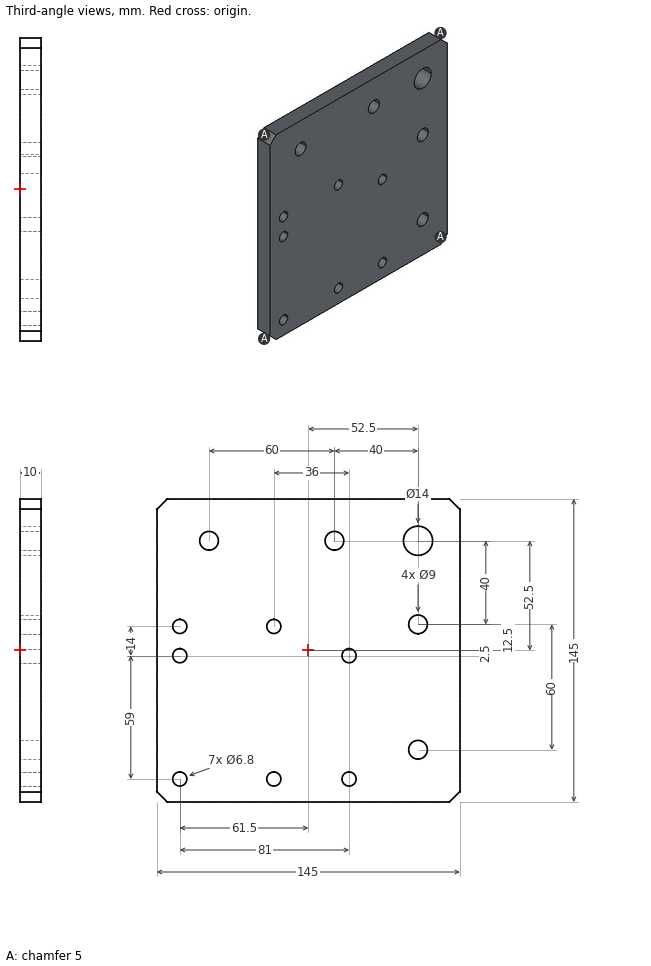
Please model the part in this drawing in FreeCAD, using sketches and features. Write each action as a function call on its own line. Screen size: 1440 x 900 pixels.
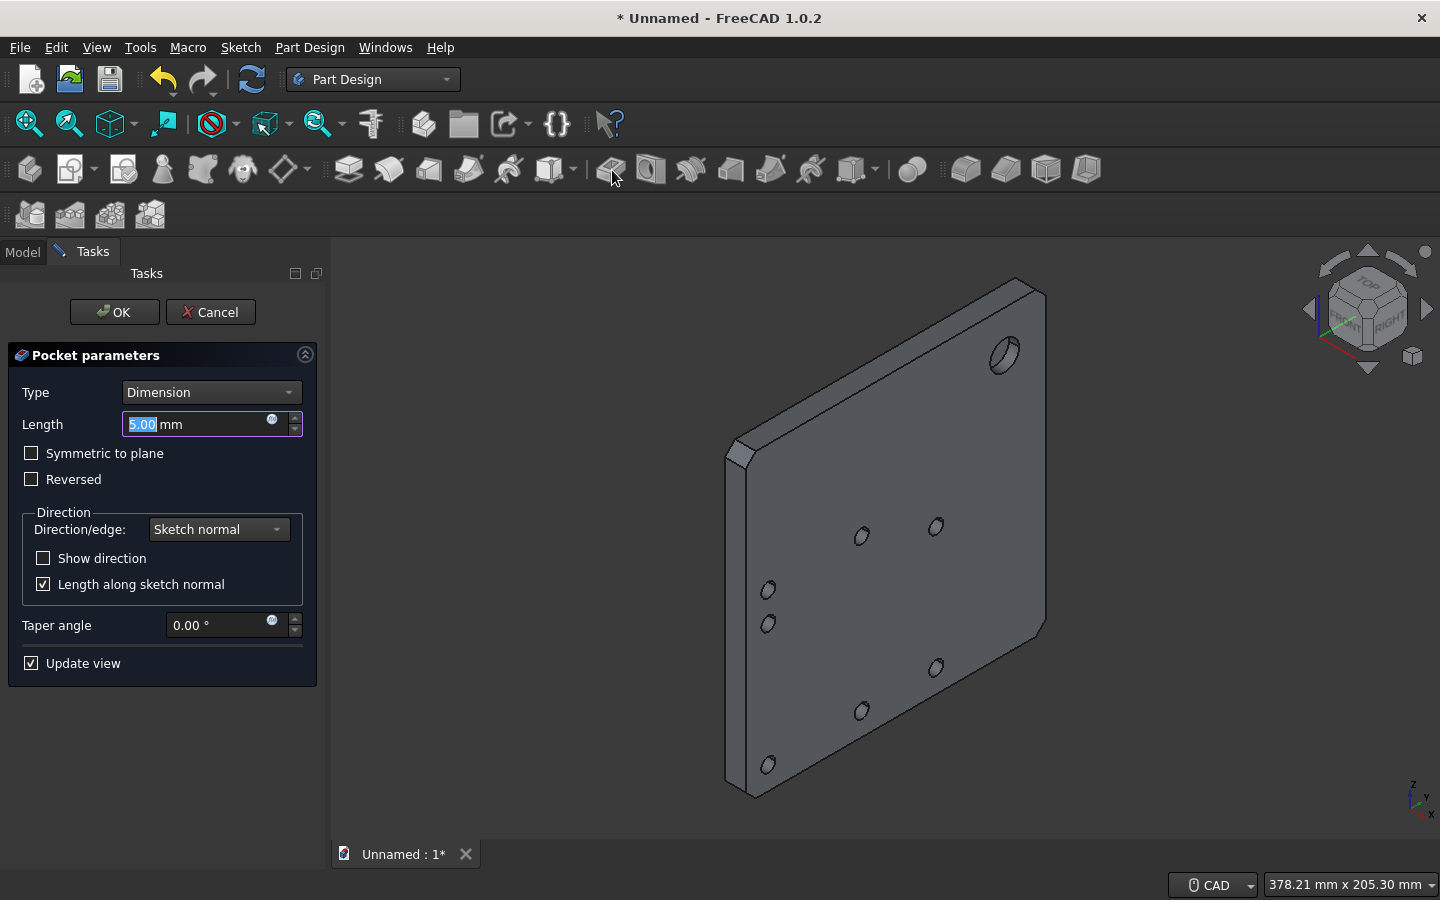
click(212, 392)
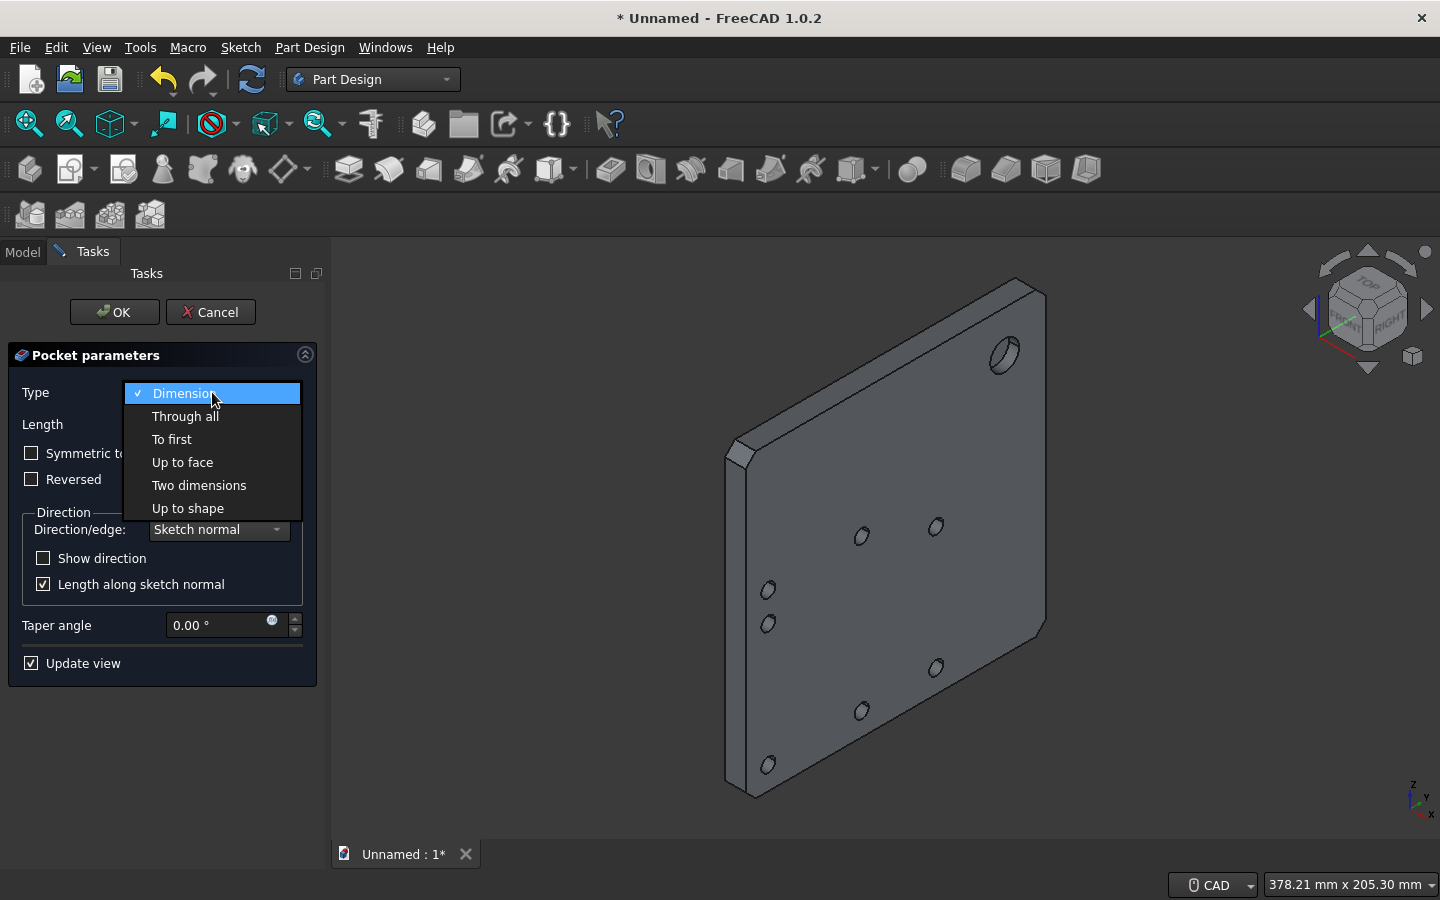
click(212, 416)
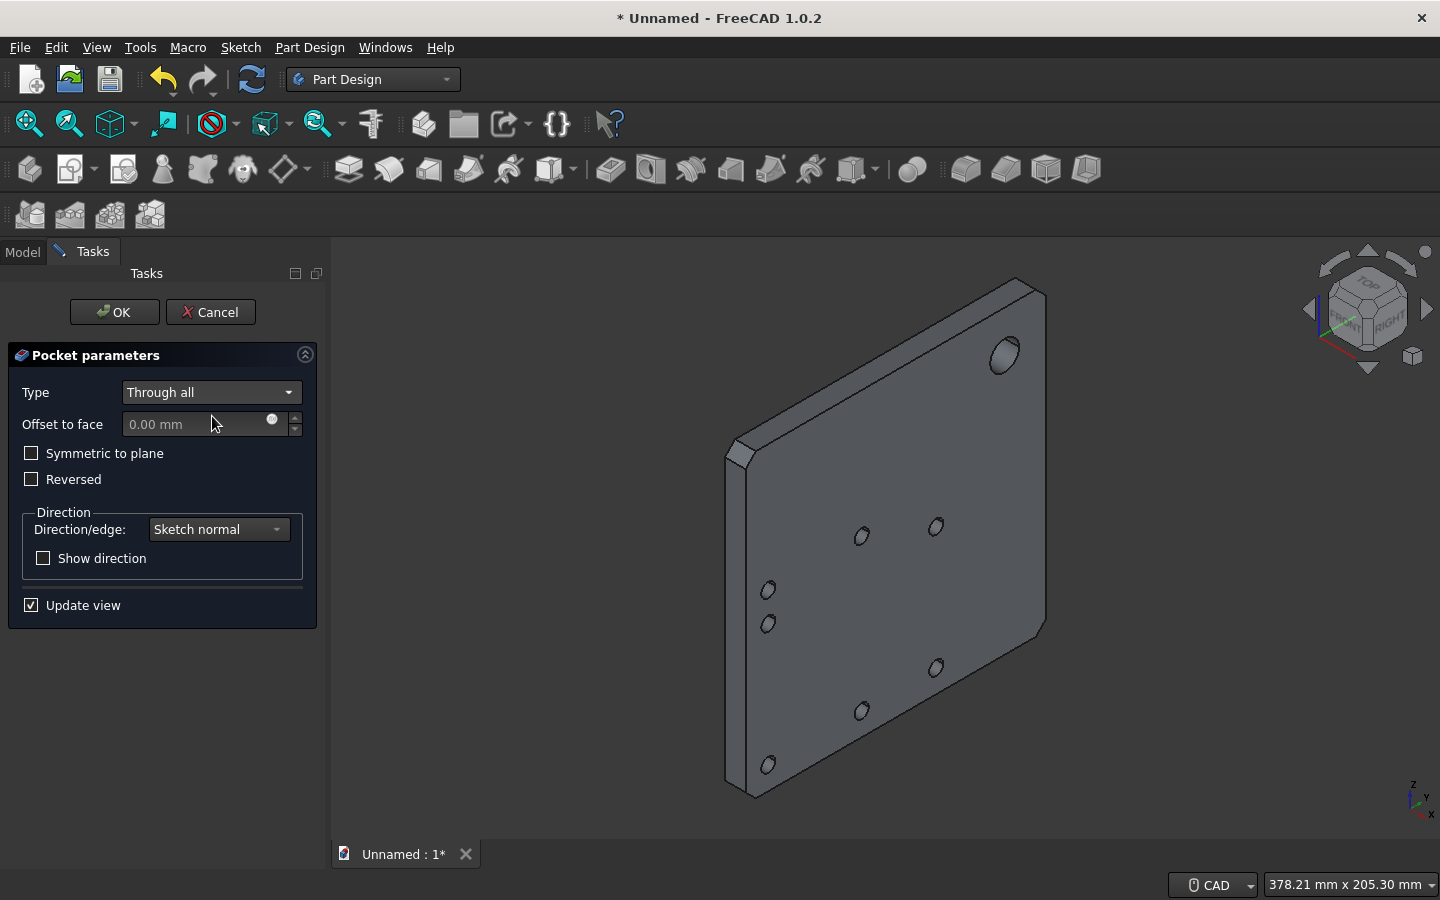
click(115, 312)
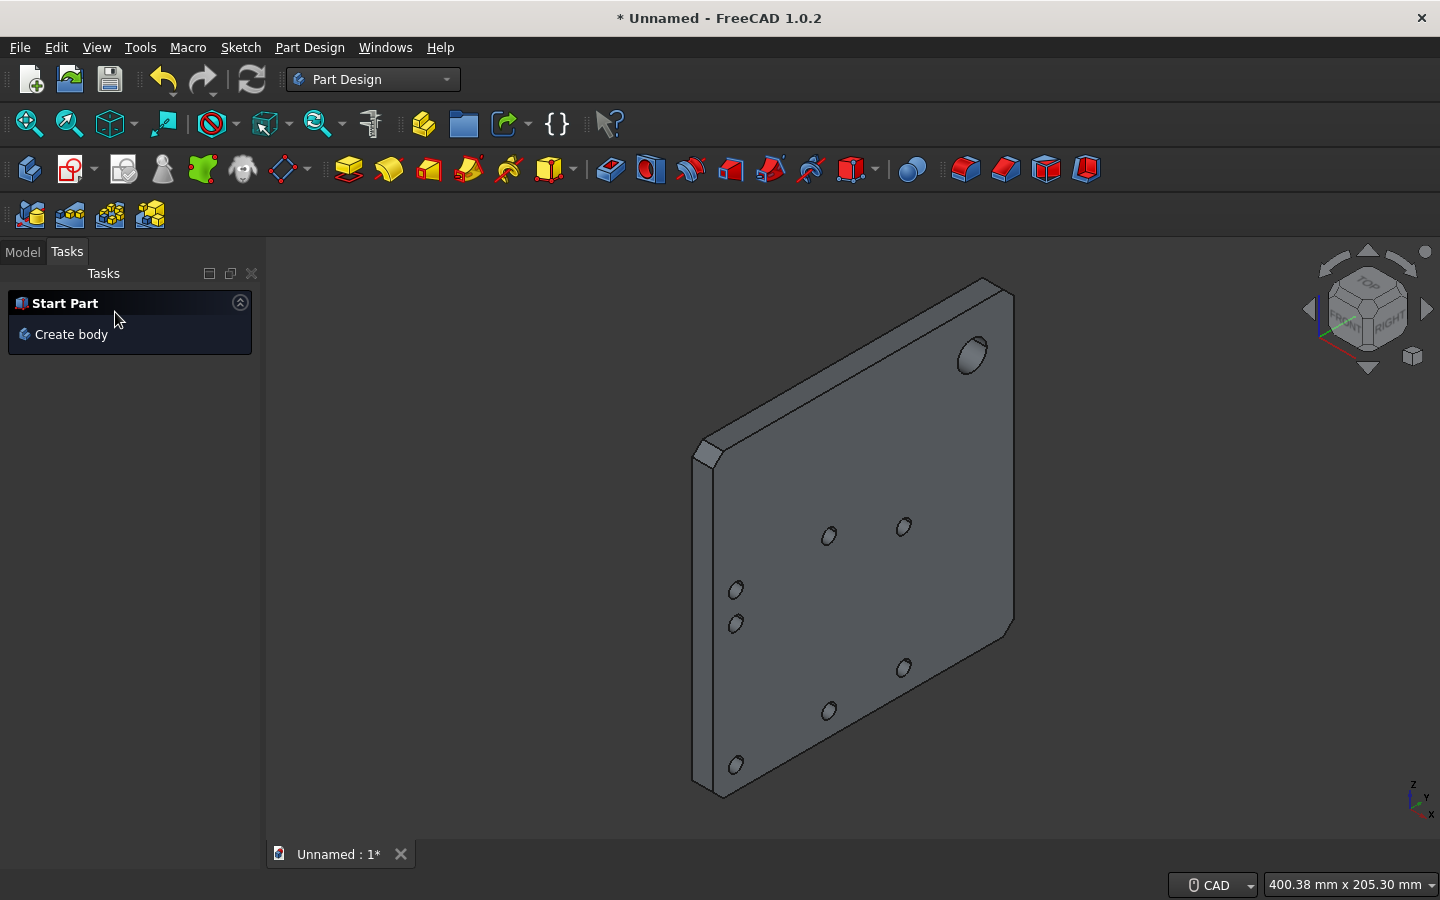
click(777, 493)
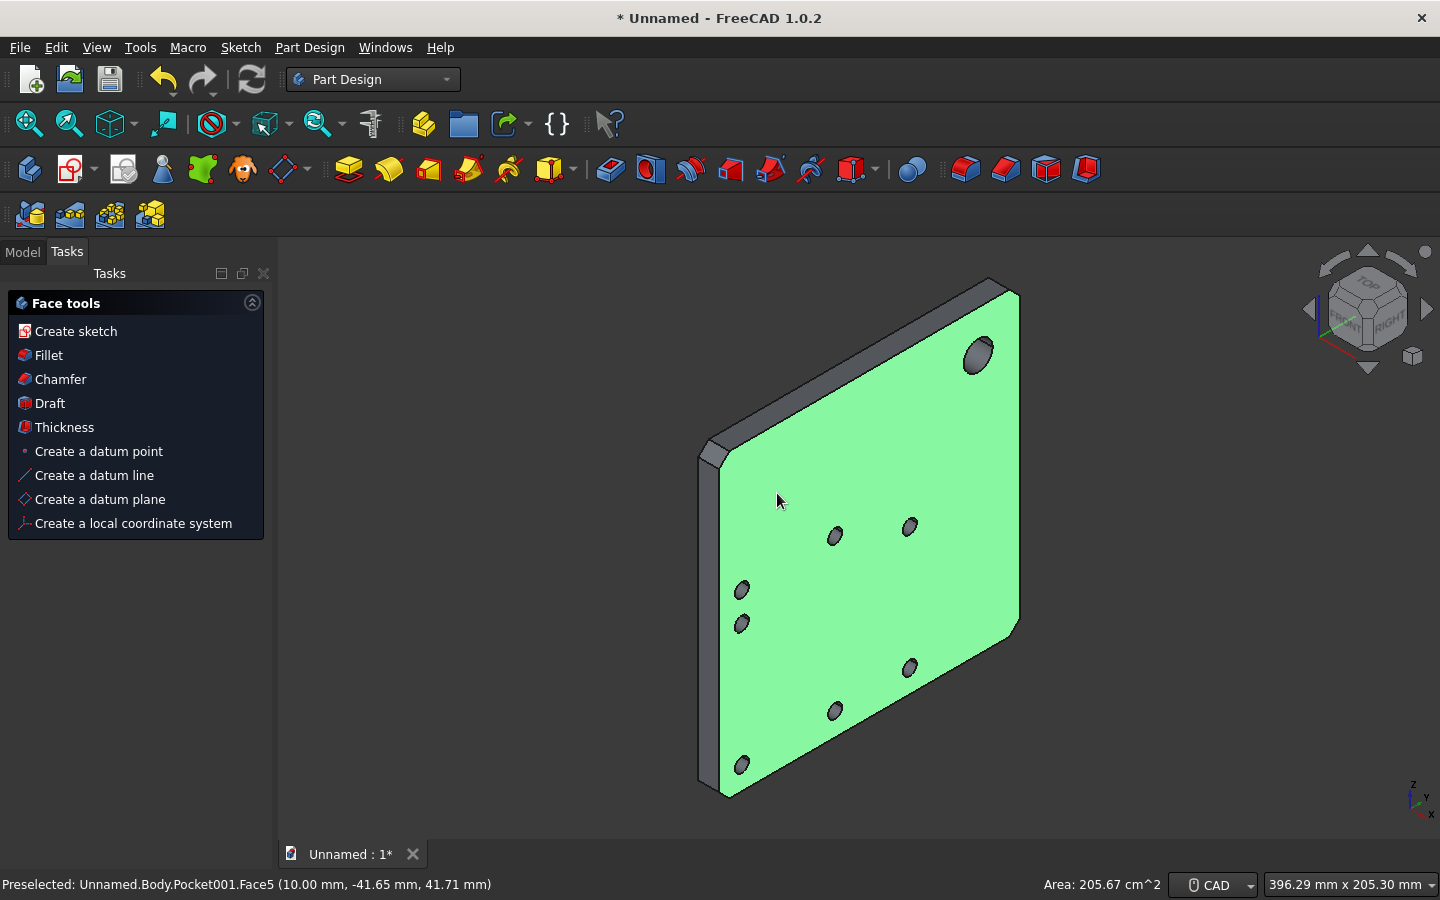
click(70, 170)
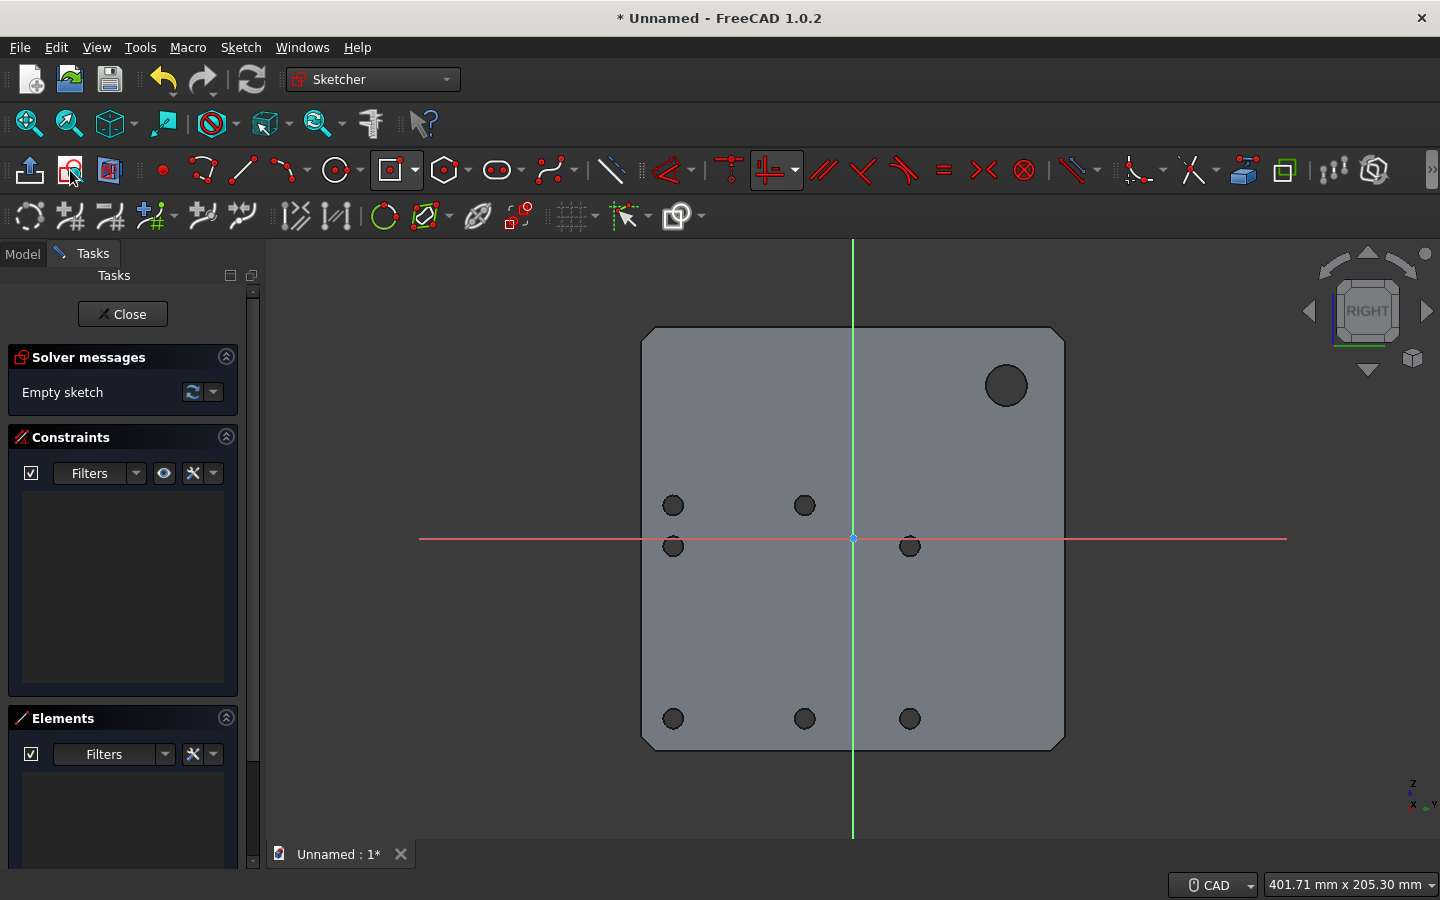
click(336, 170)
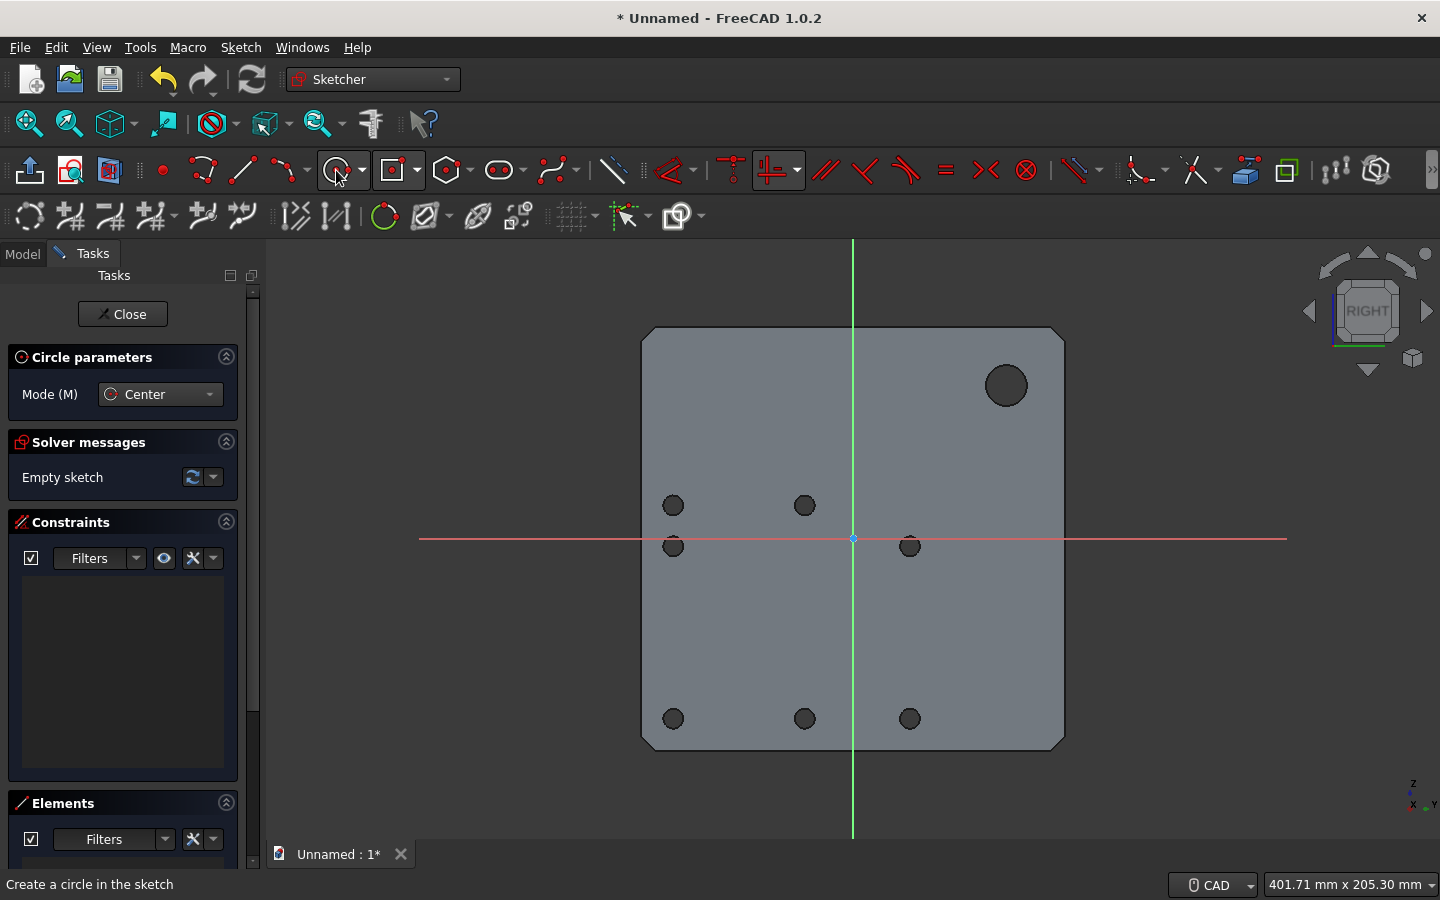
scroll(1006, 502, up, 3)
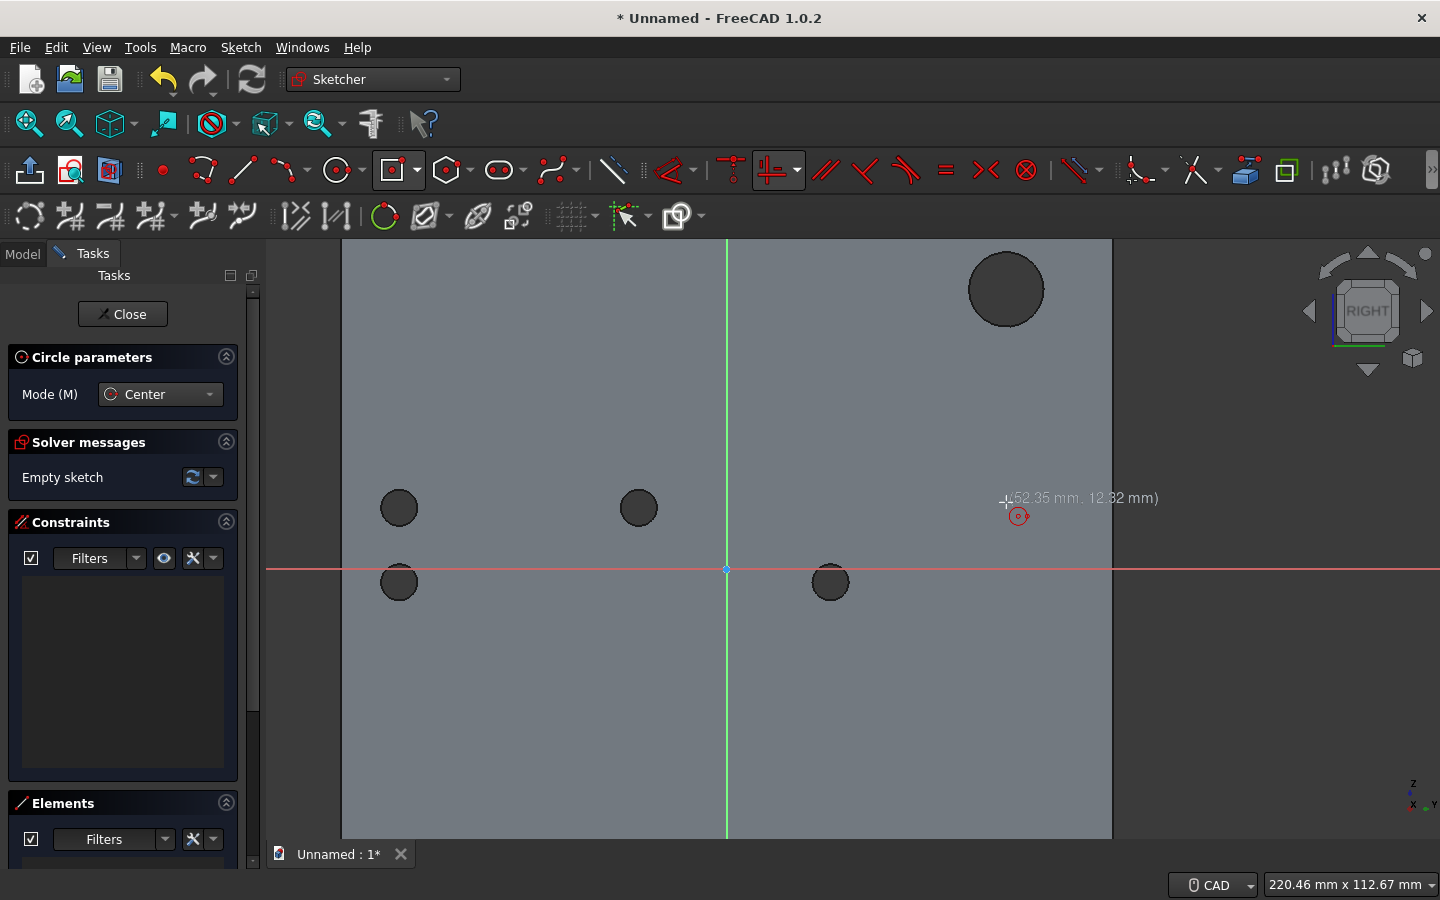
click(1006, 502)
click(1023, 486)